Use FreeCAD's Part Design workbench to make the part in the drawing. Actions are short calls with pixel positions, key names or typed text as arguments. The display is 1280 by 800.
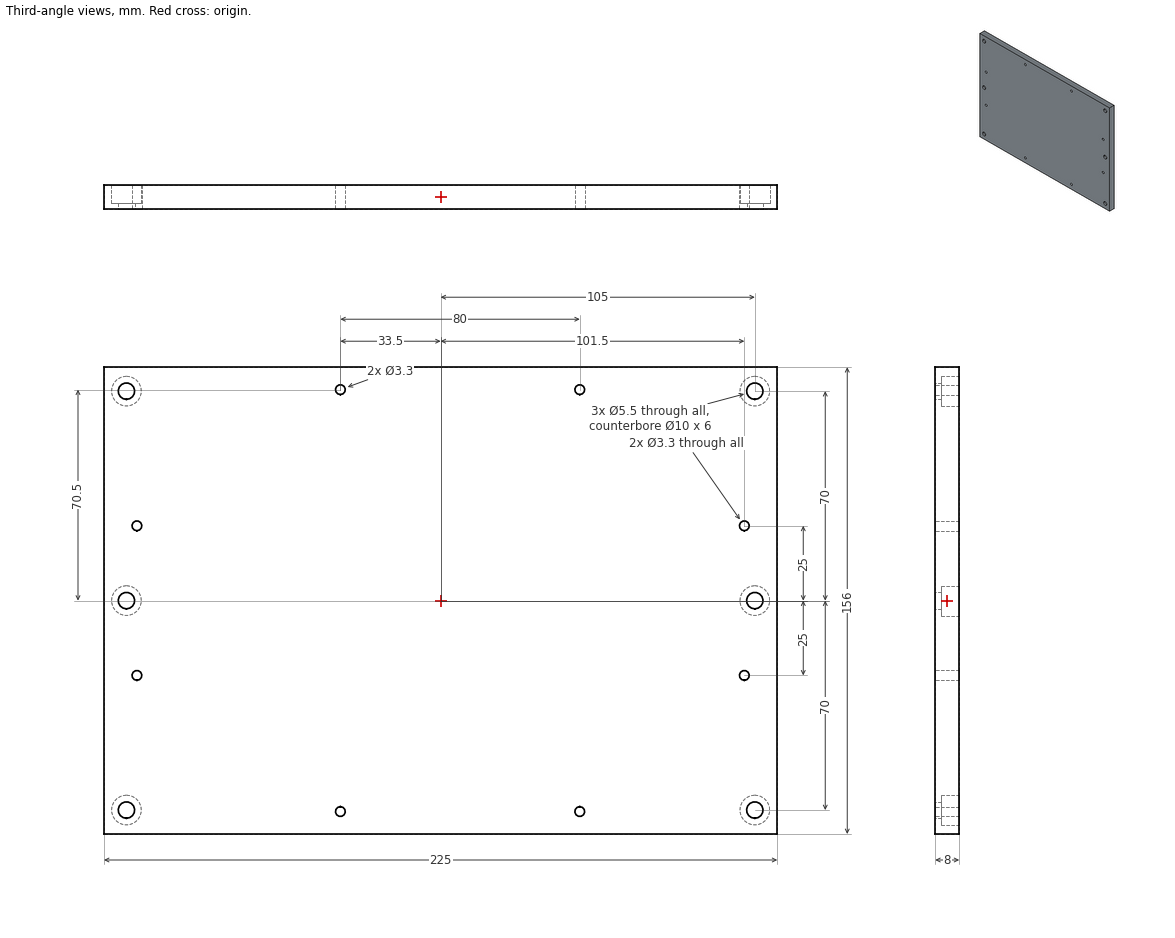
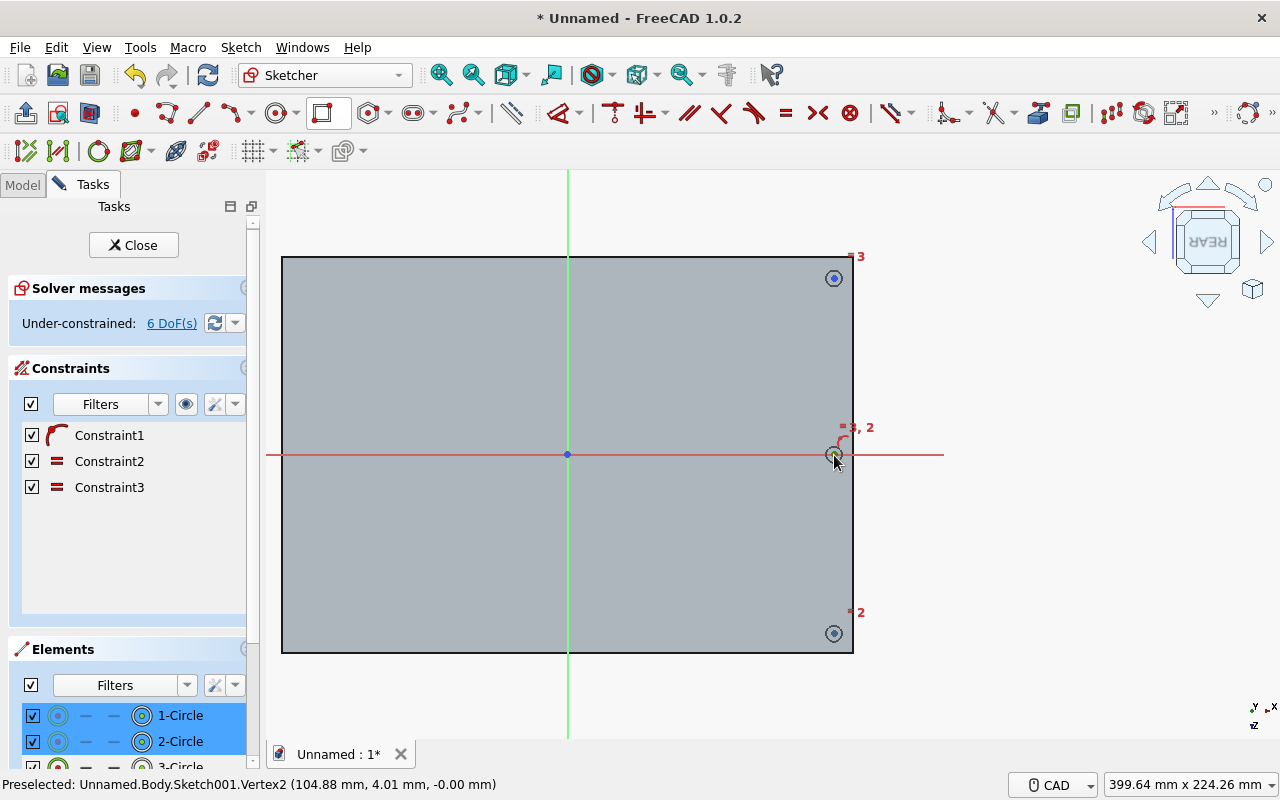
key(v)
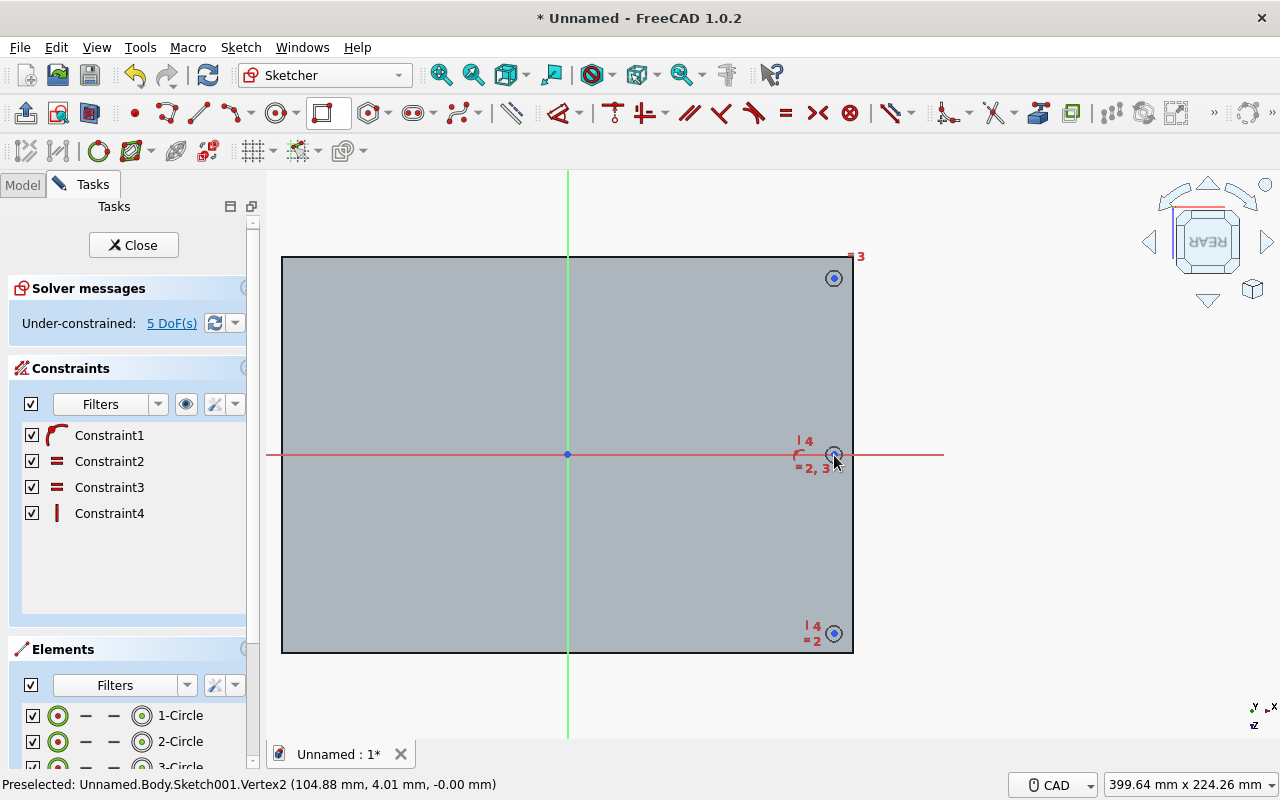
click(834, 455)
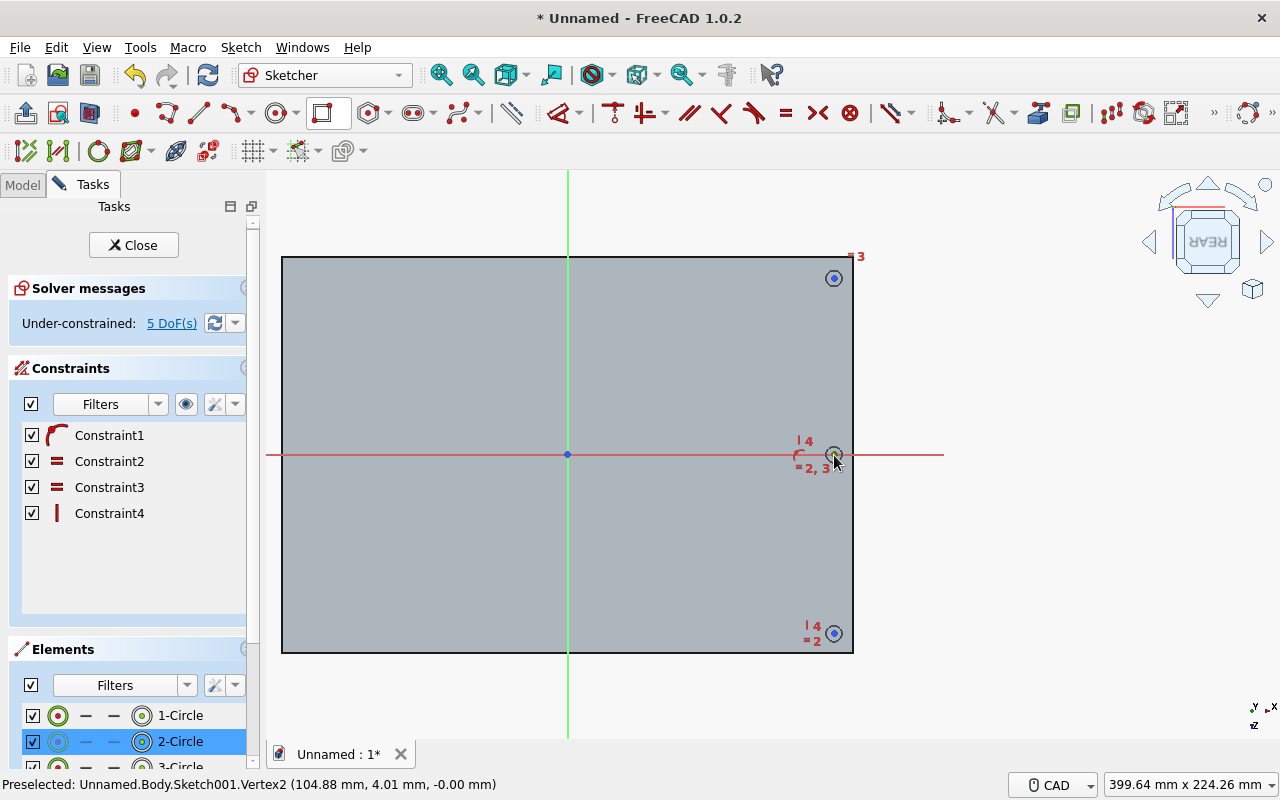
click(834, 278)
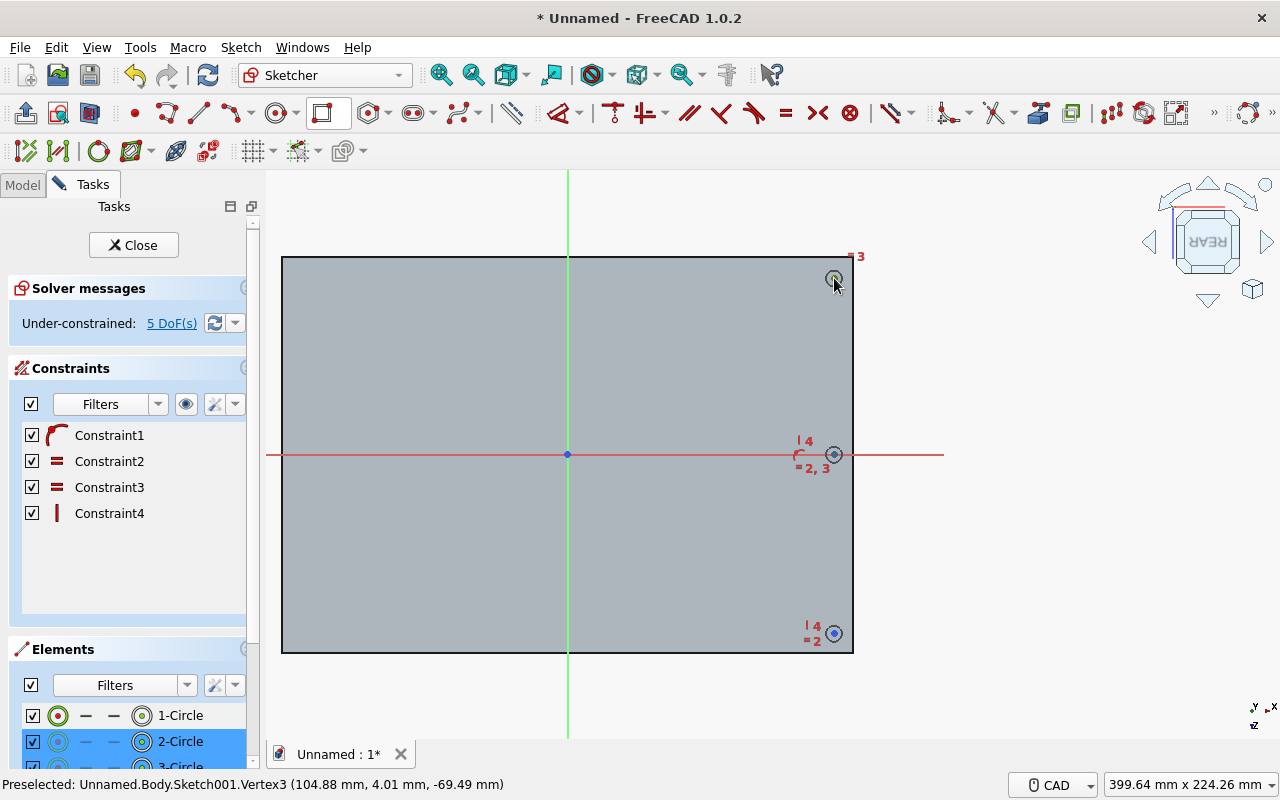
key(v)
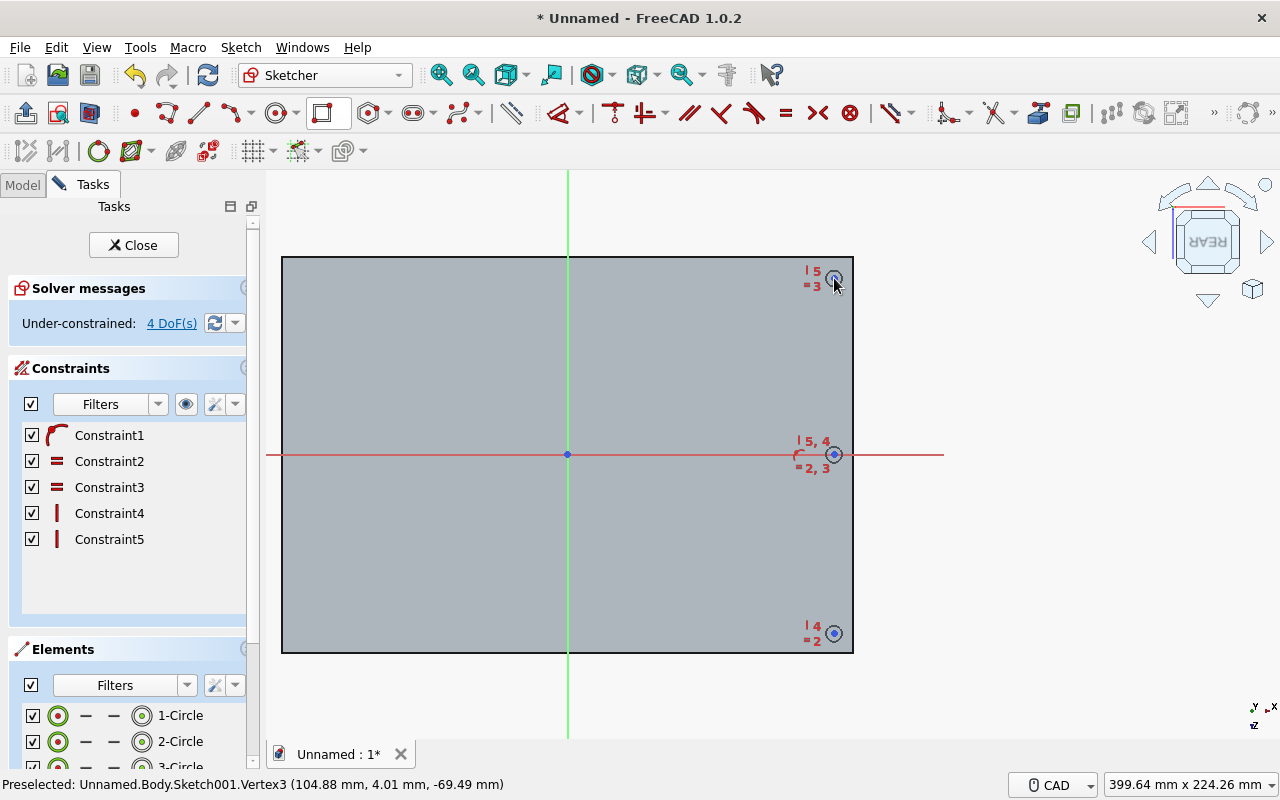
key(d)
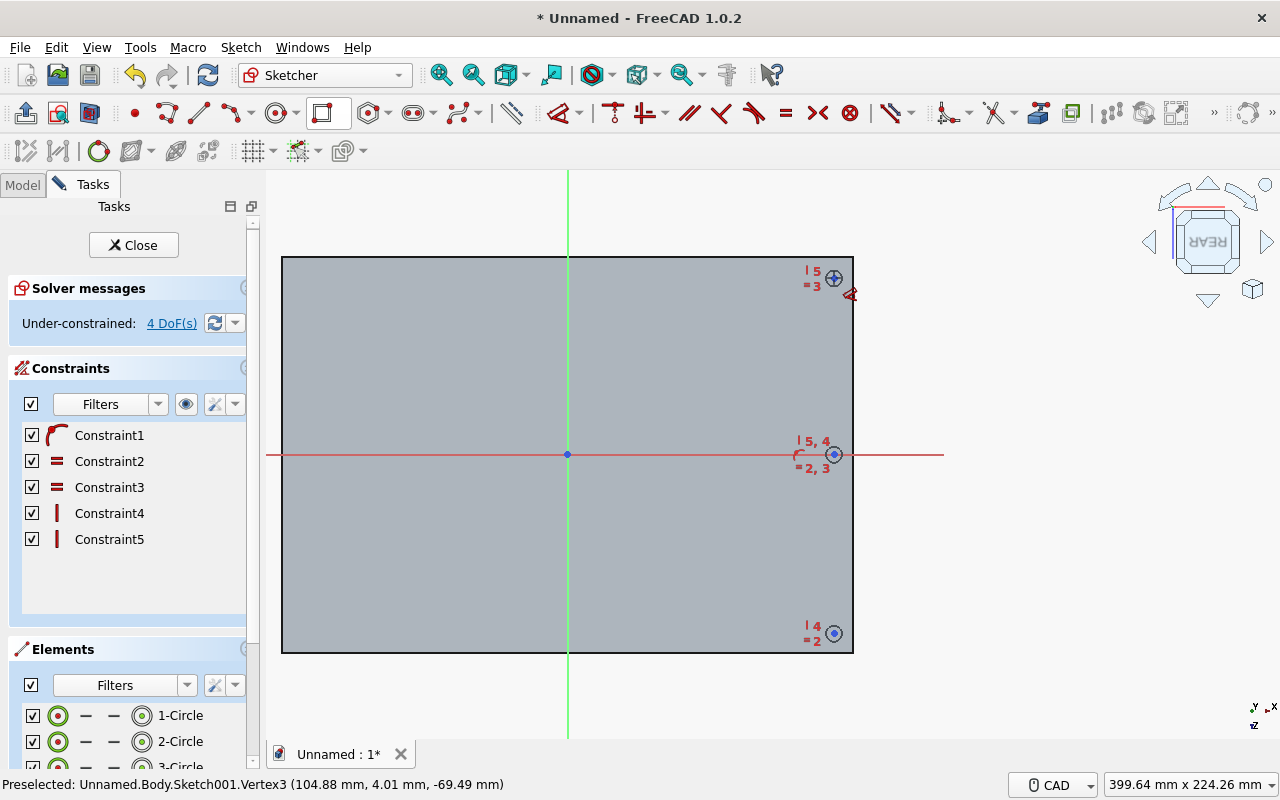
scroll(826, 634, up, 6)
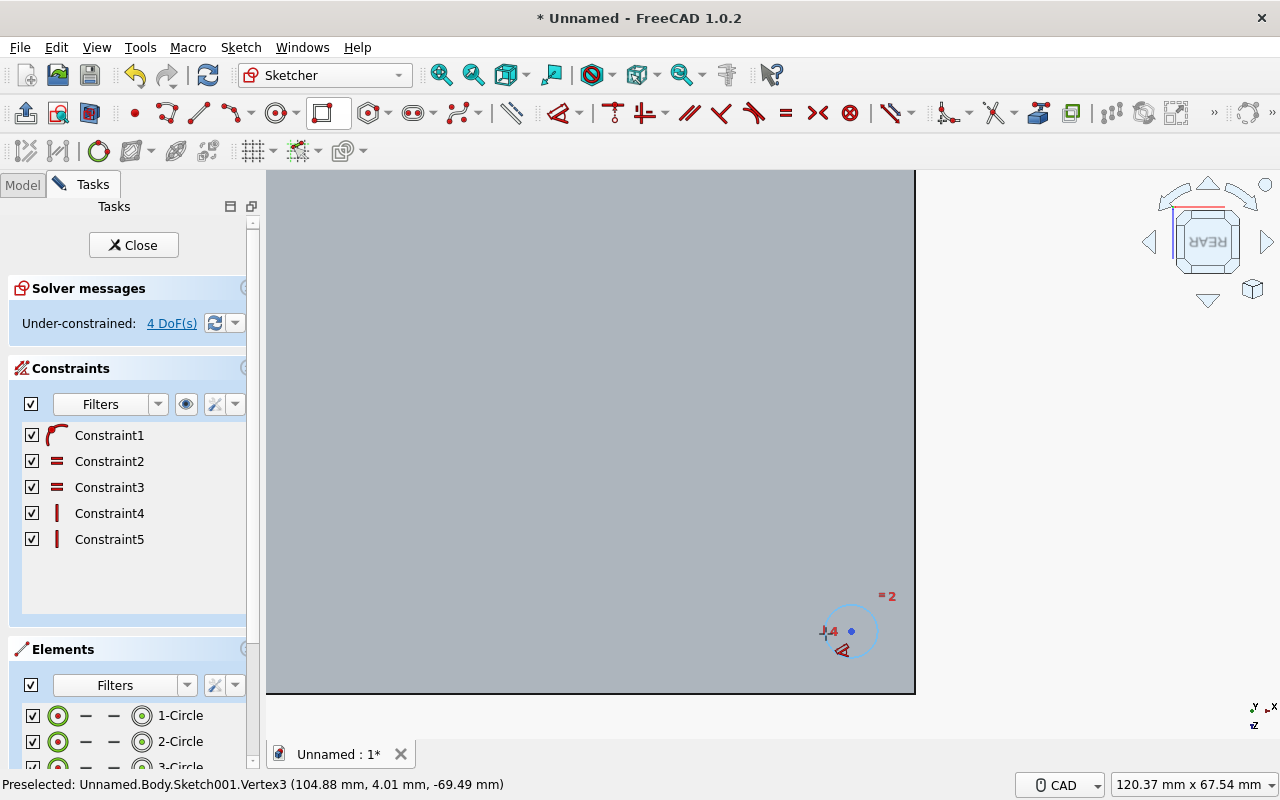
click(825, 631)
click(793, 631)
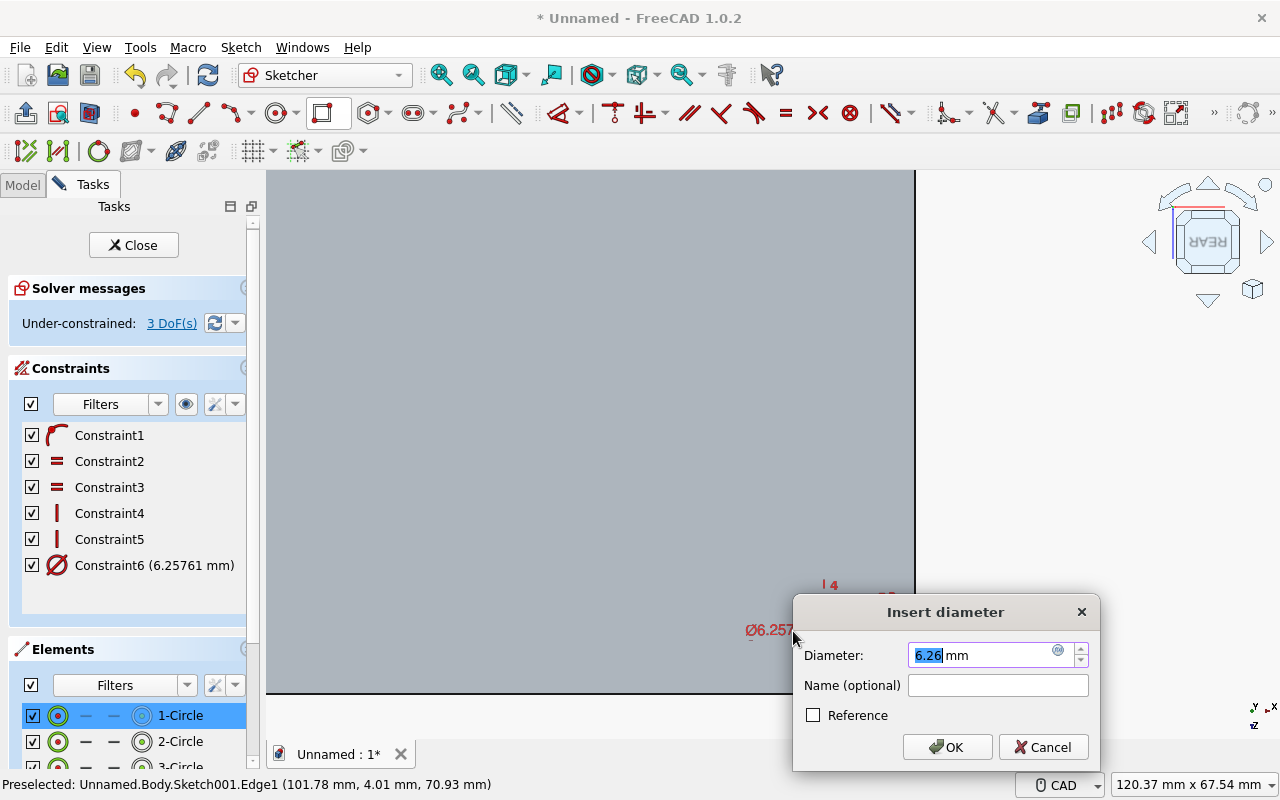
text(5.5)
key(Return)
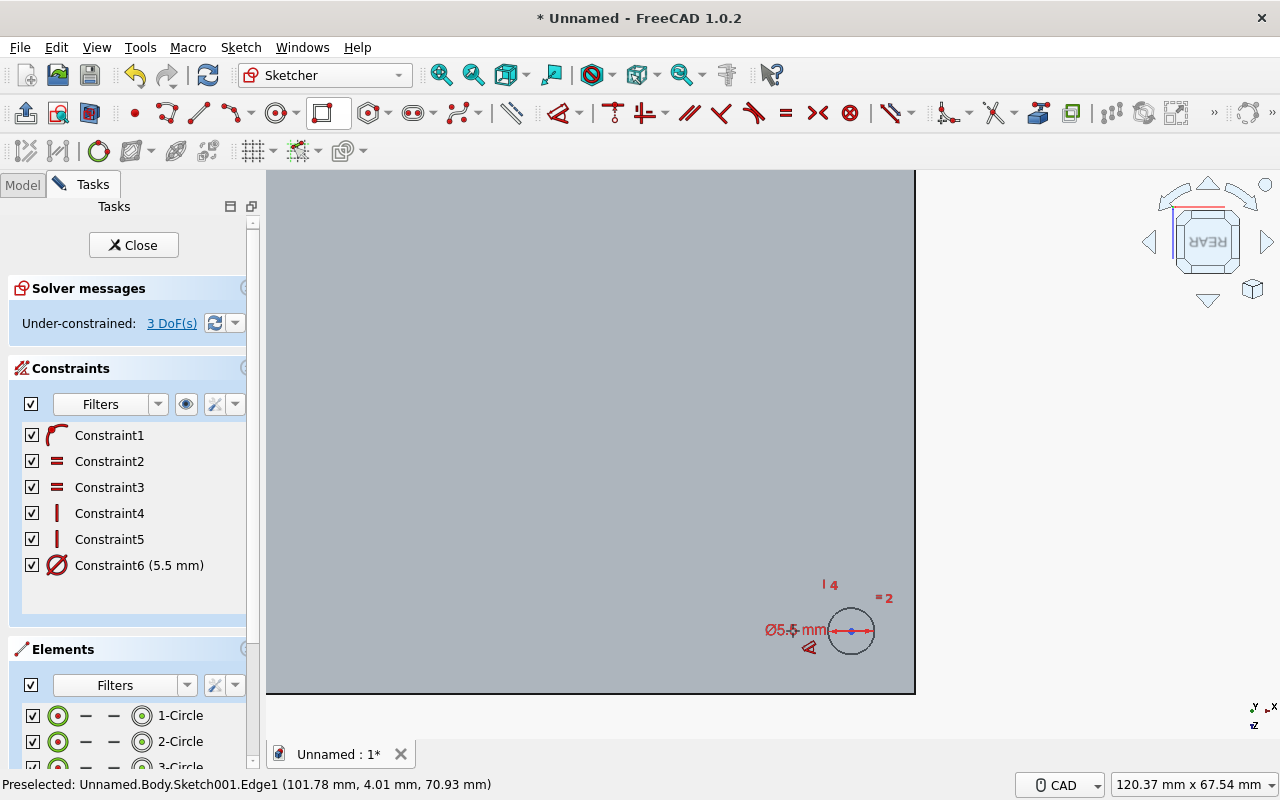
scroll(826, 634, down, 6)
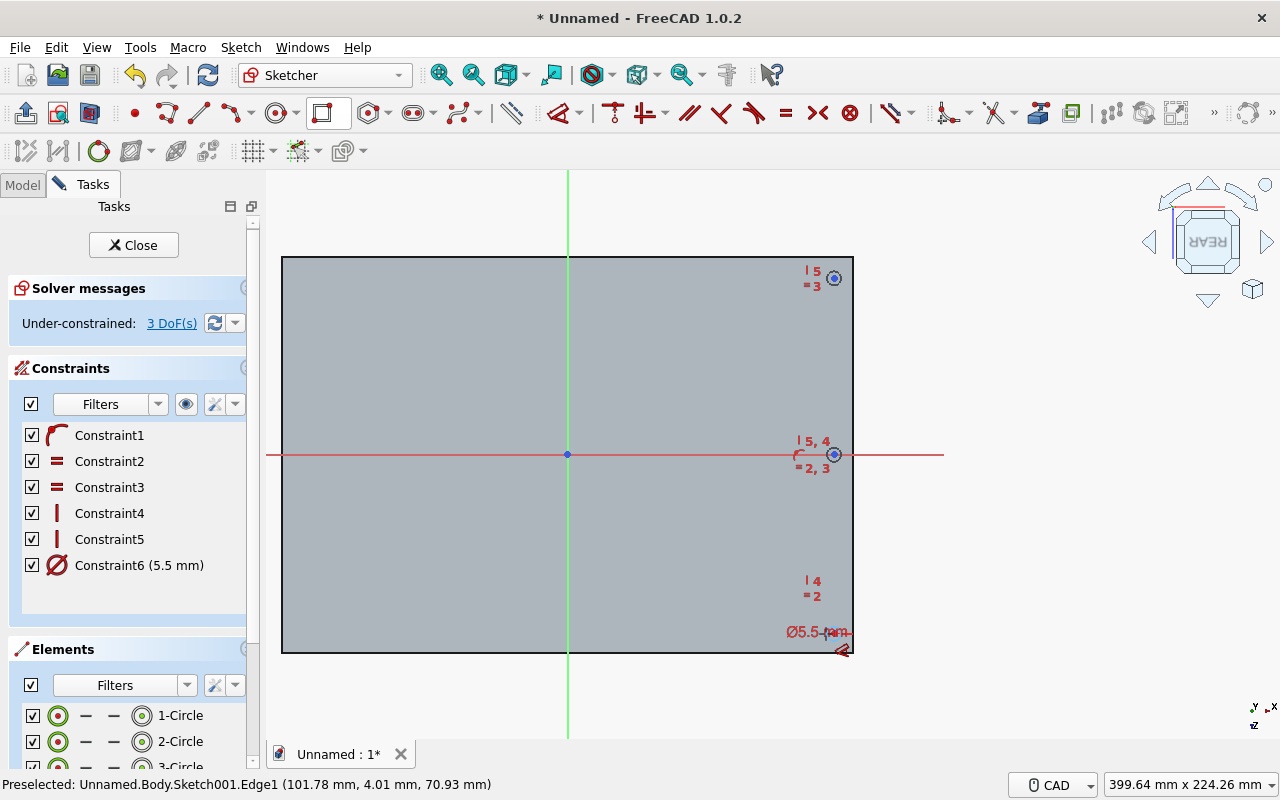
click(834, 634)
click(534, 544)